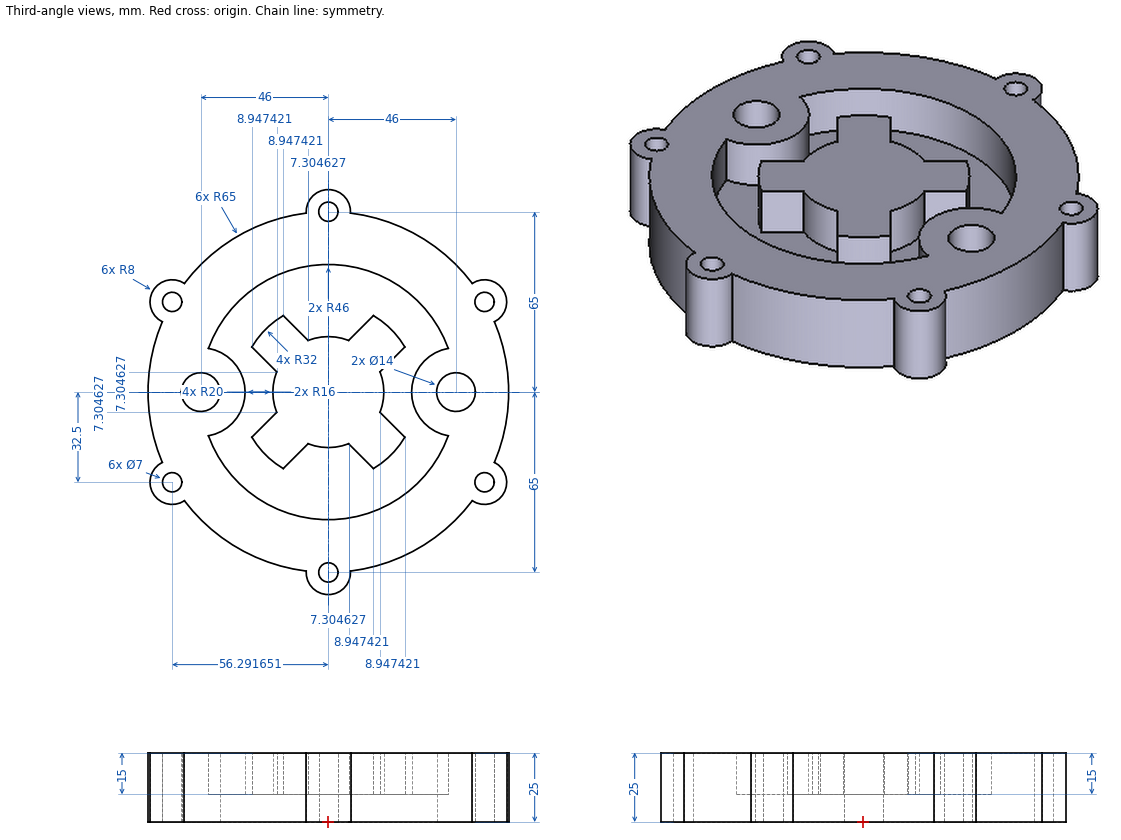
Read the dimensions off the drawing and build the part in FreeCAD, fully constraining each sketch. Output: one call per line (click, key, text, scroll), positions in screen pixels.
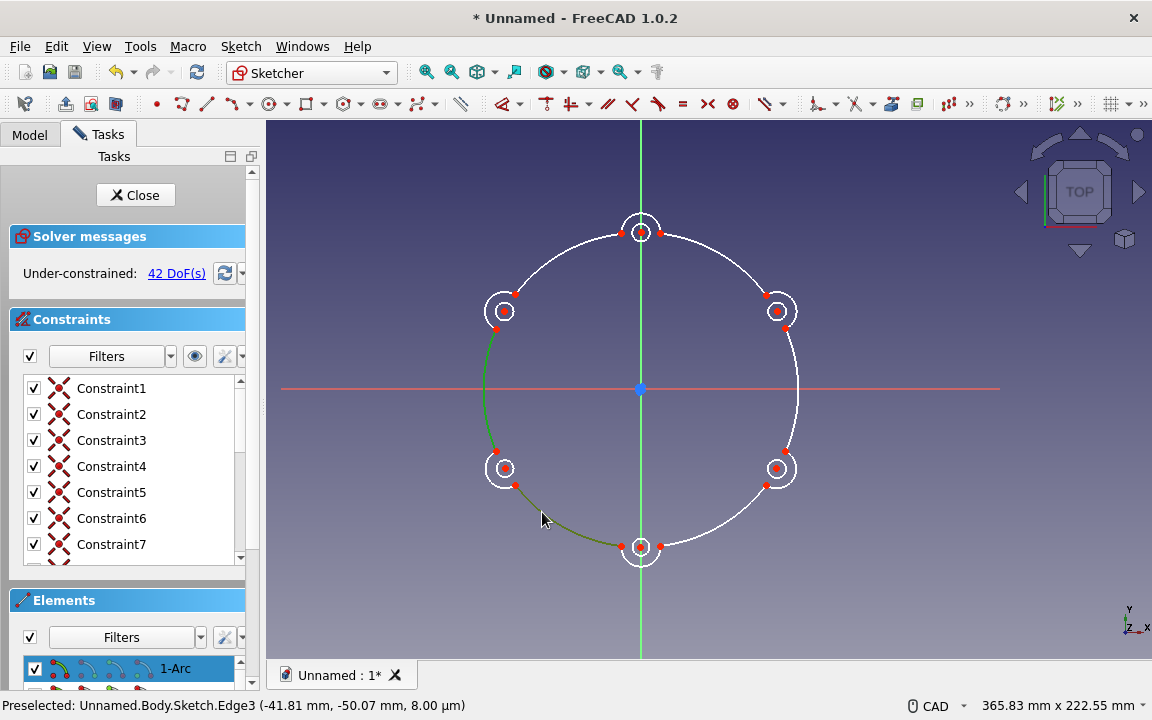
click(546, 104)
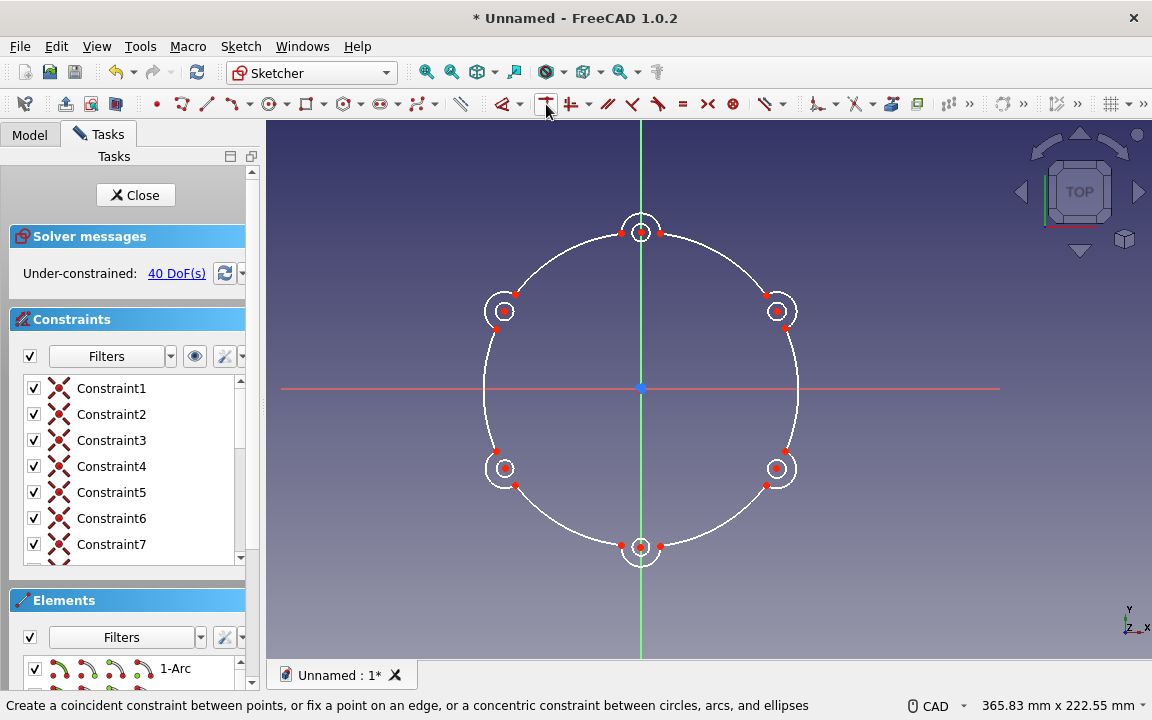
click(486, 365)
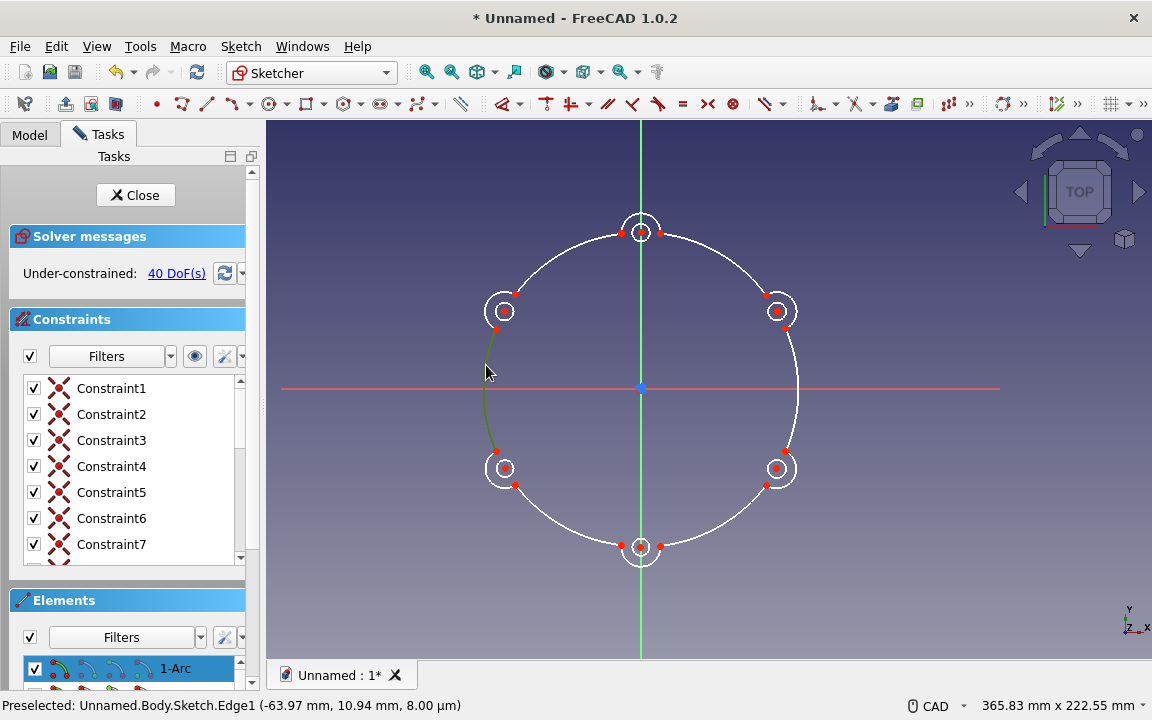
click(697, 537)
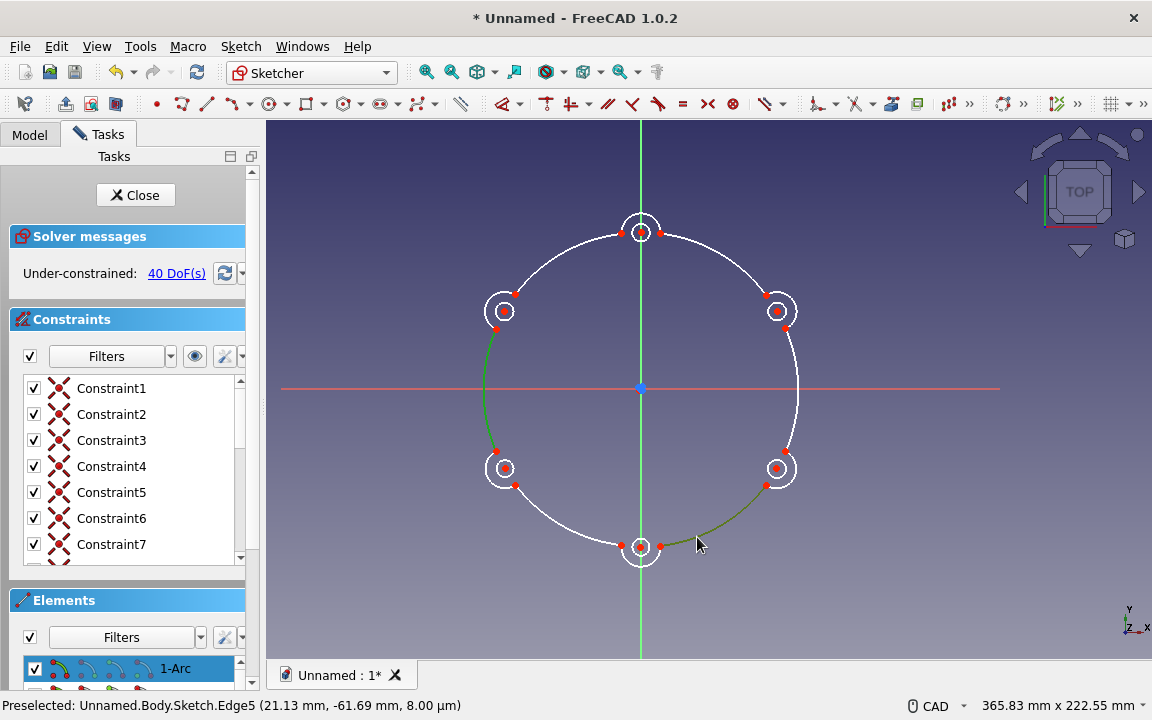
click(546, 104)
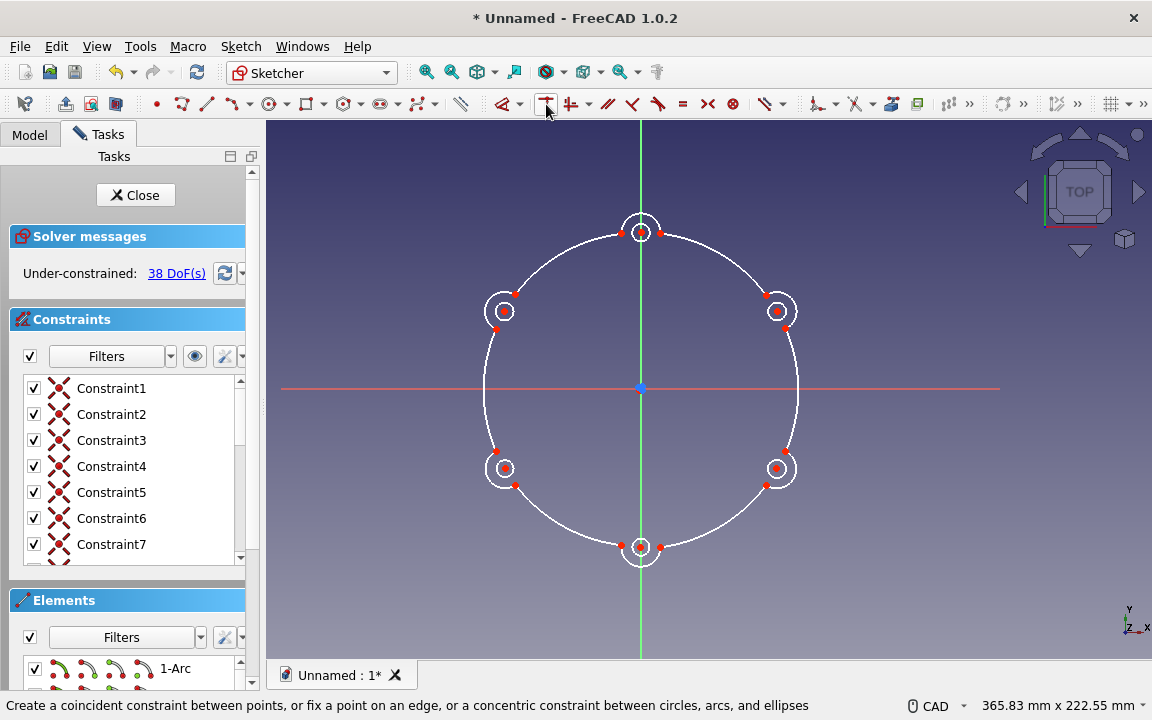
click(486, 365)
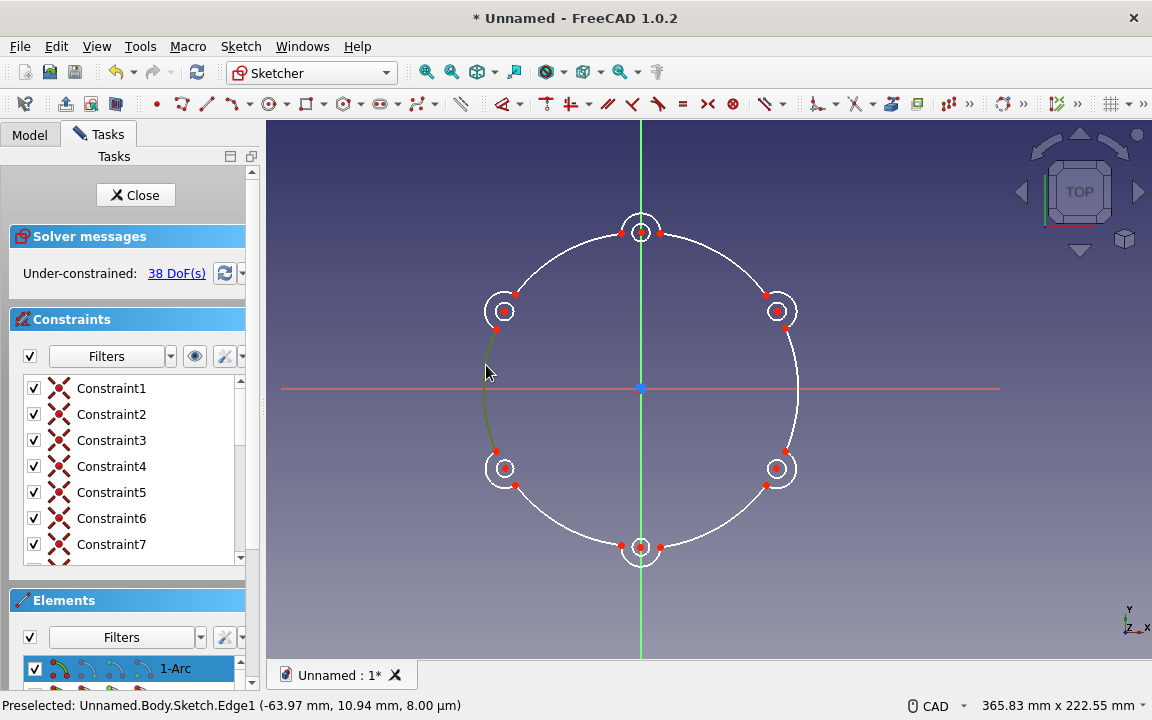
click(796, 415)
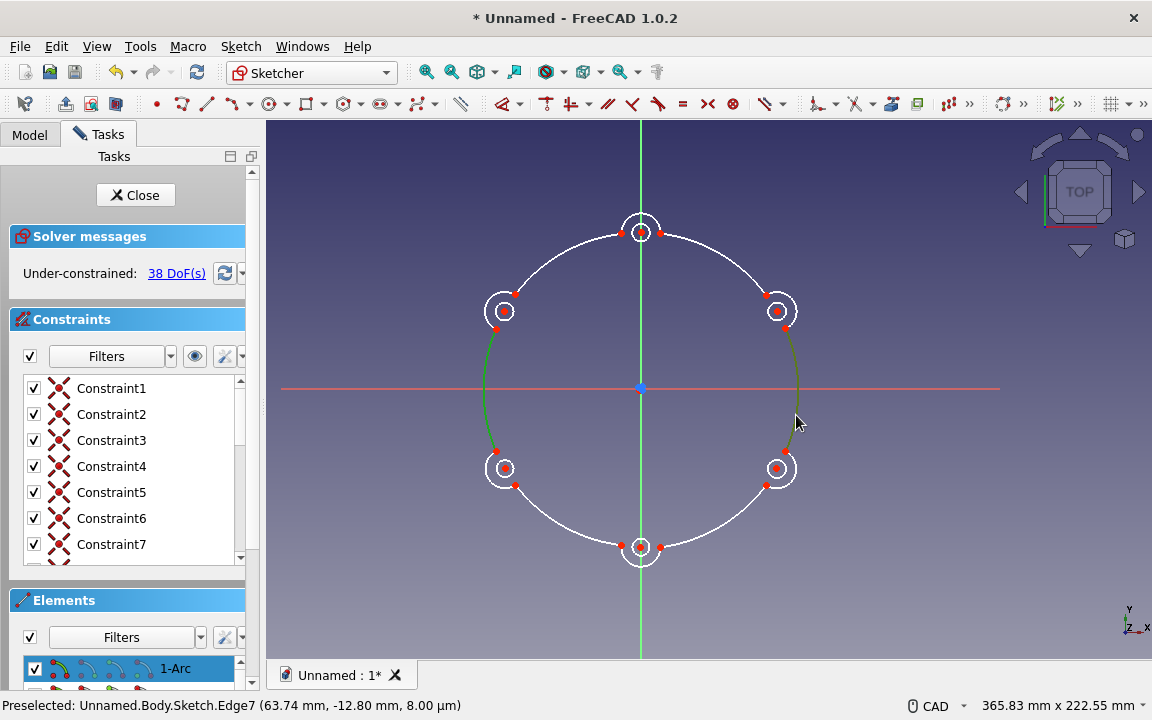
click(546, 104)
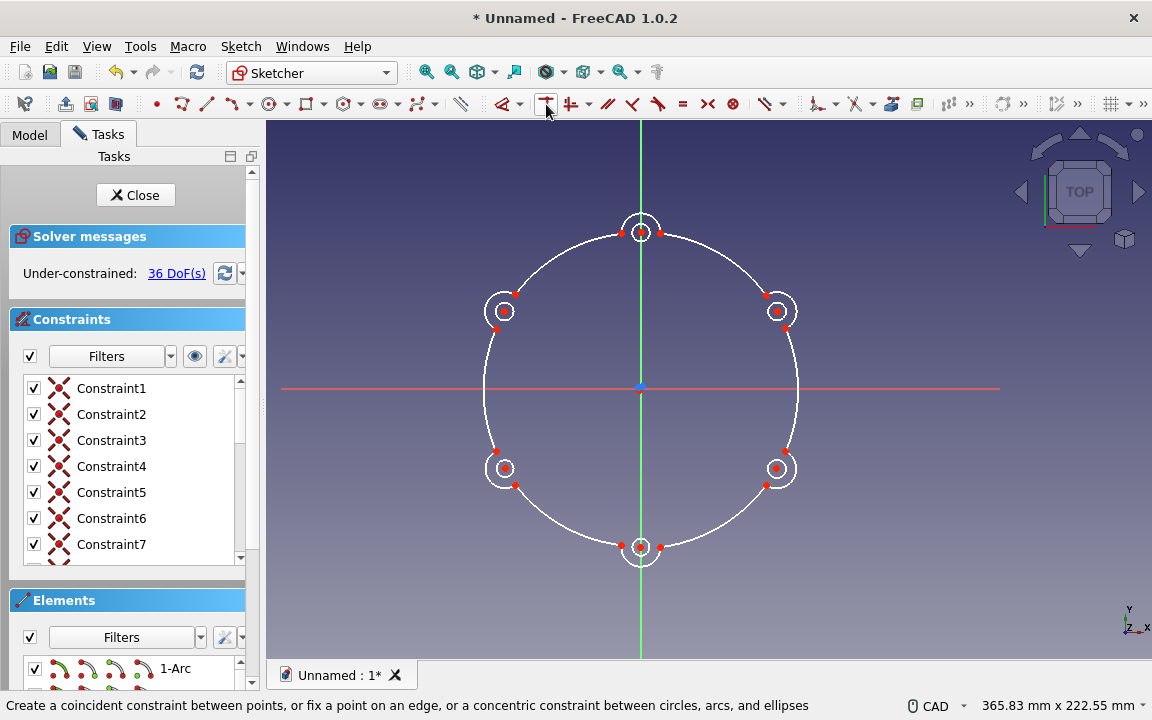
click(486, 365)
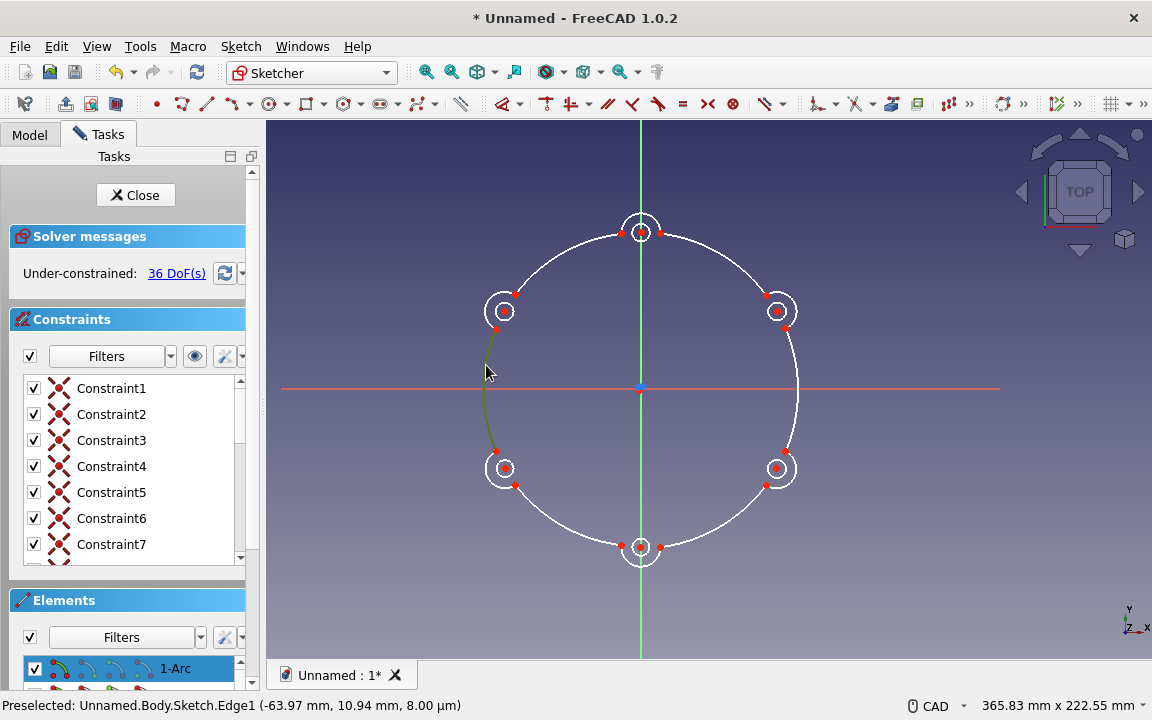
click(740, 268)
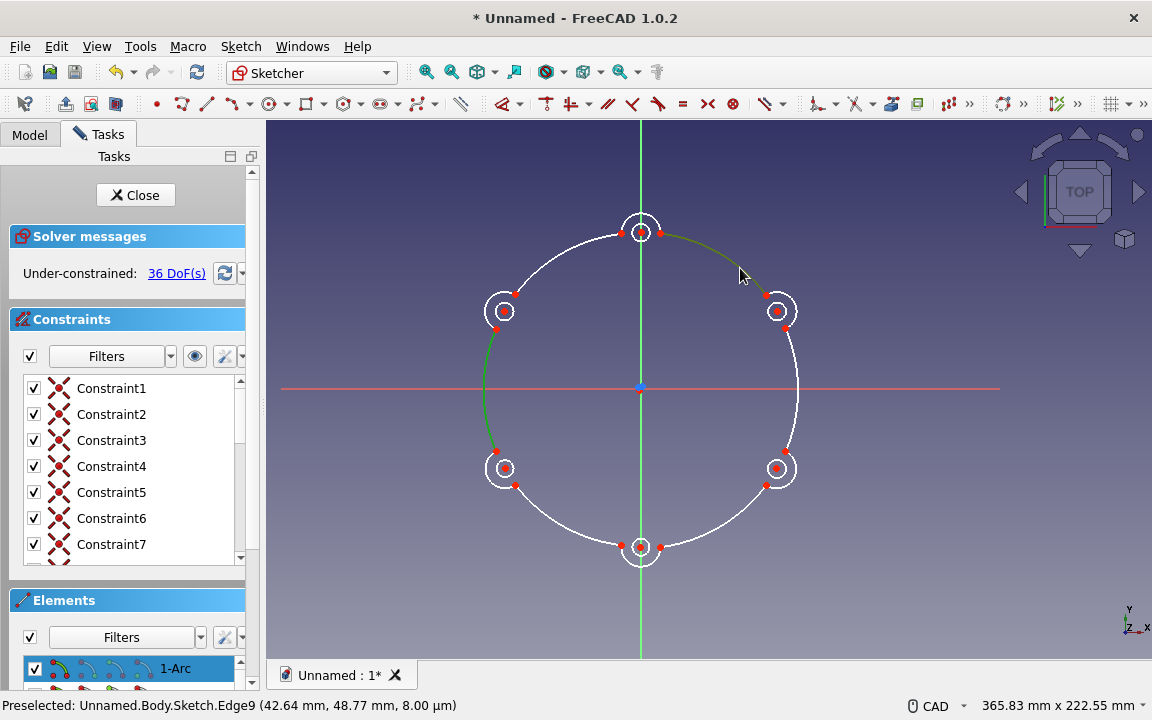
click(546, 104)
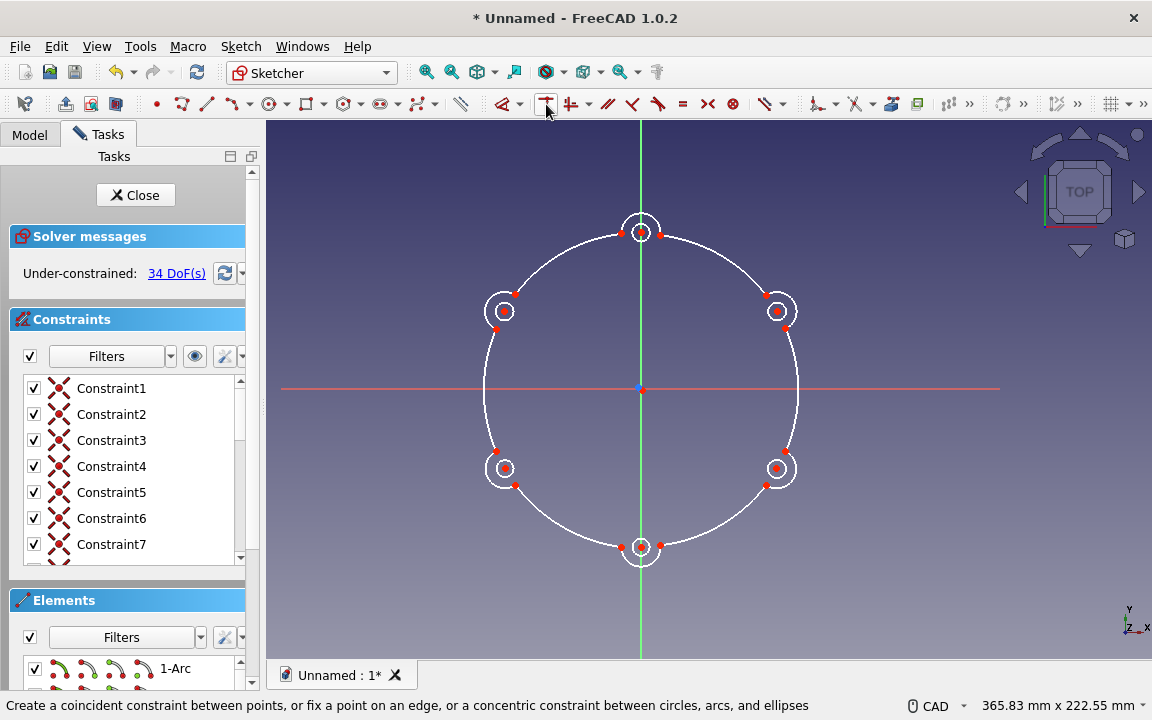
click(486, 365)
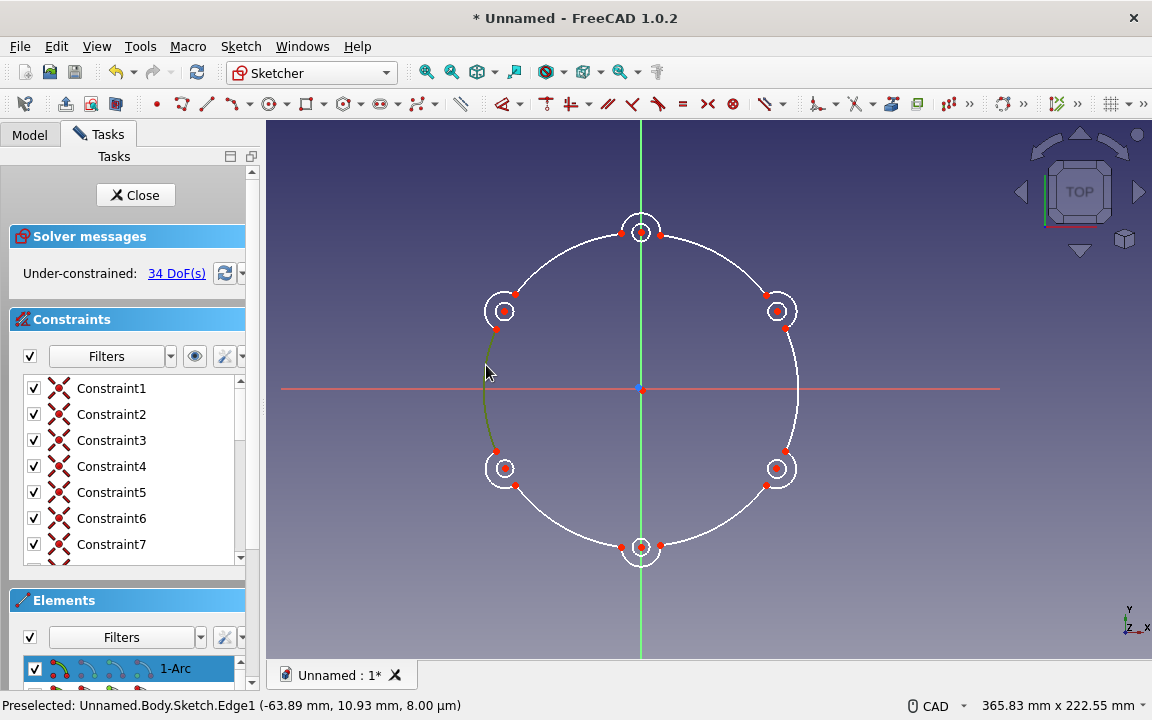
click(585, 243)